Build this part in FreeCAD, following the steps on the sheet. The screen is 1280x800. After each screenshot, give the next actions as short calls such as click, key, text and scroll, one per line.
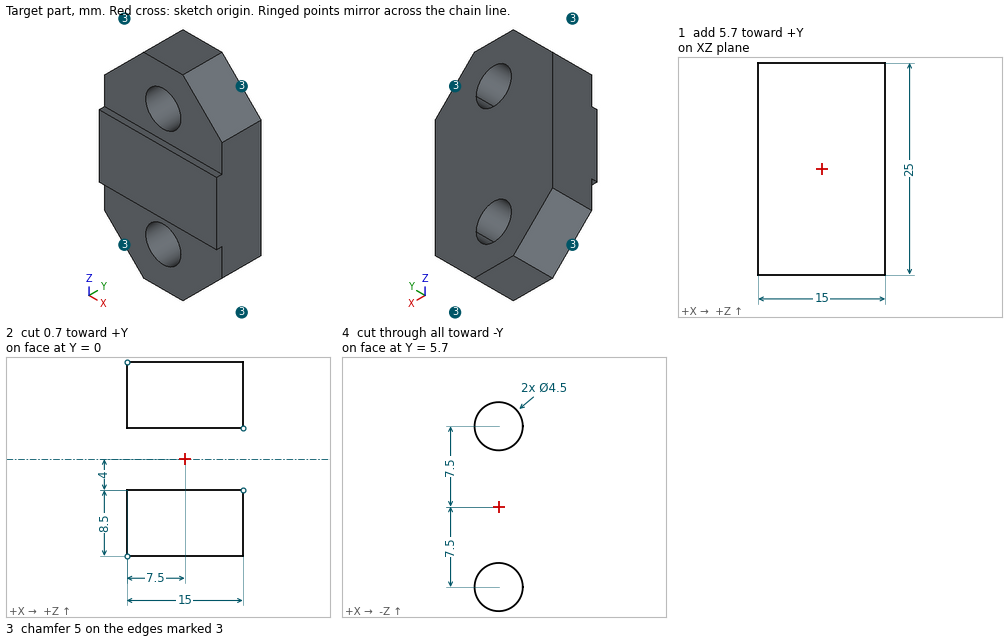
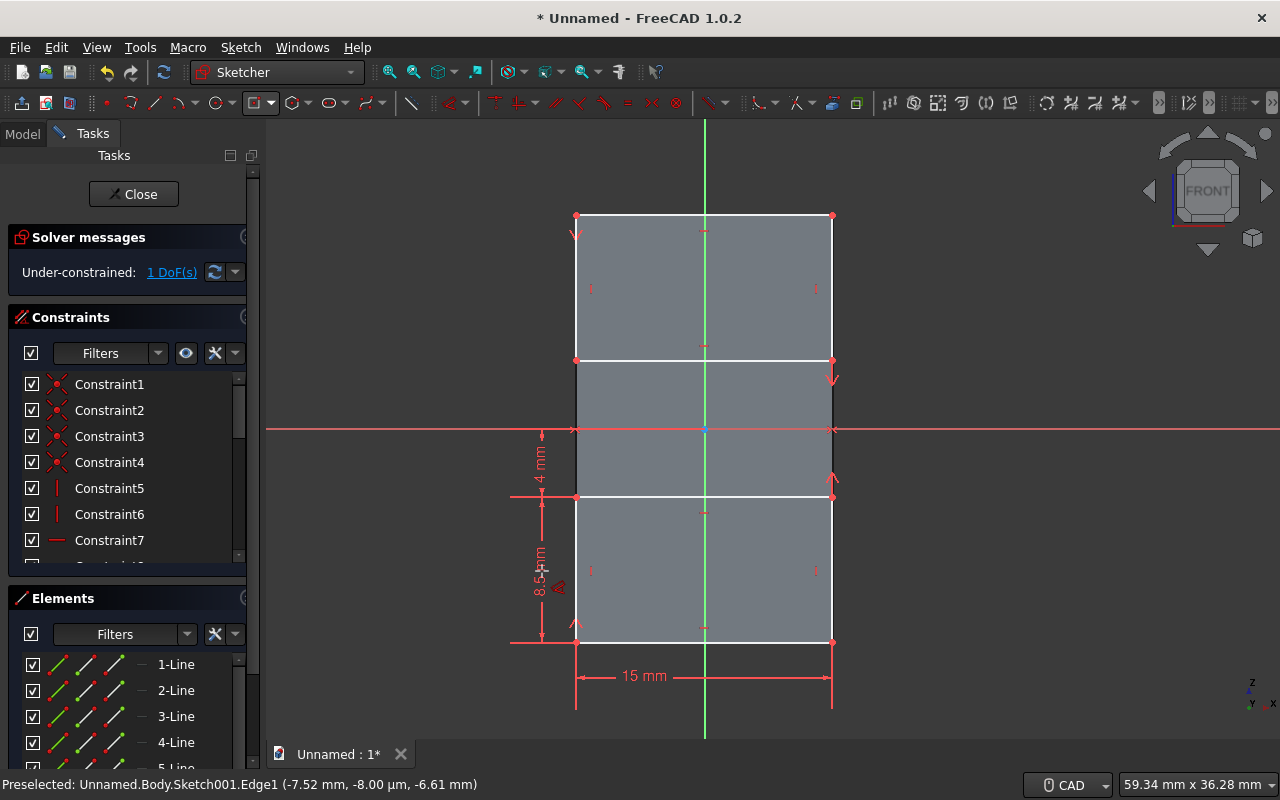
click(576, 497)
click(640, 531)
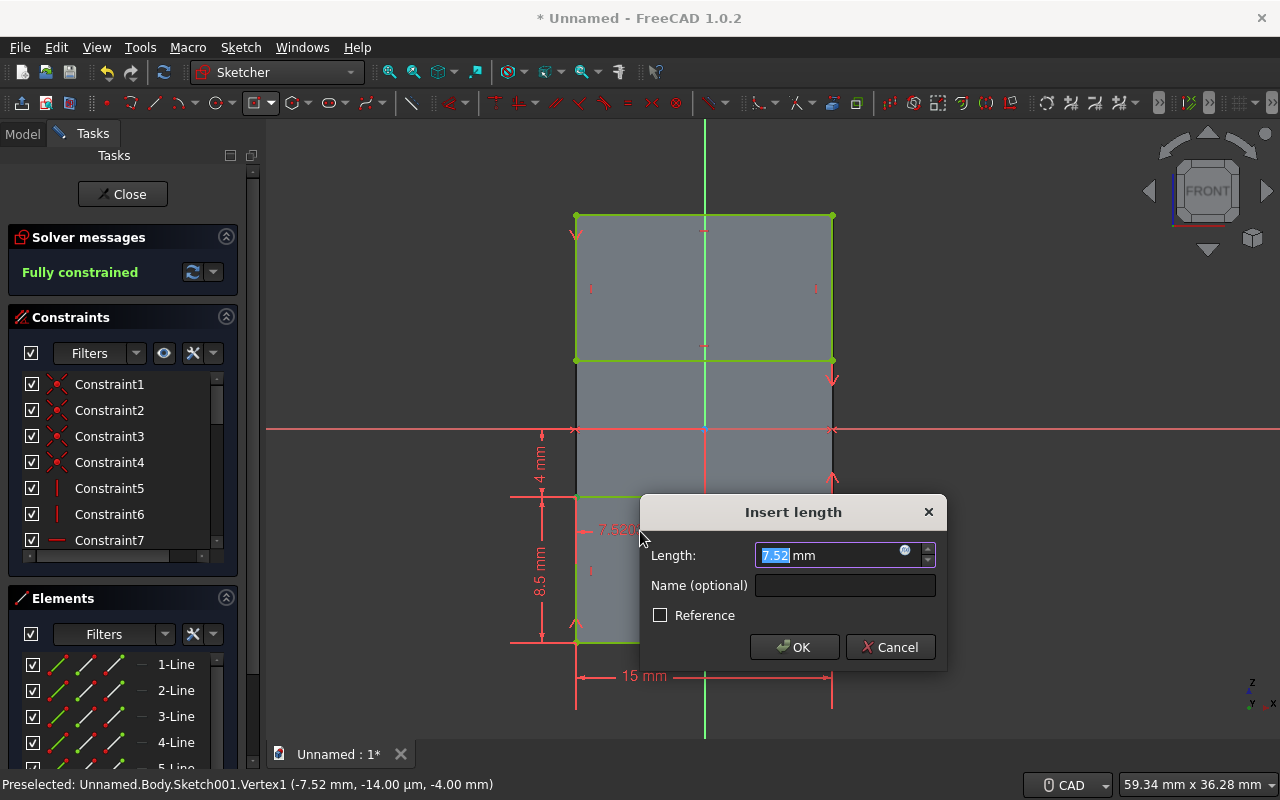
text(7.5)
key(Return)
key(Escape)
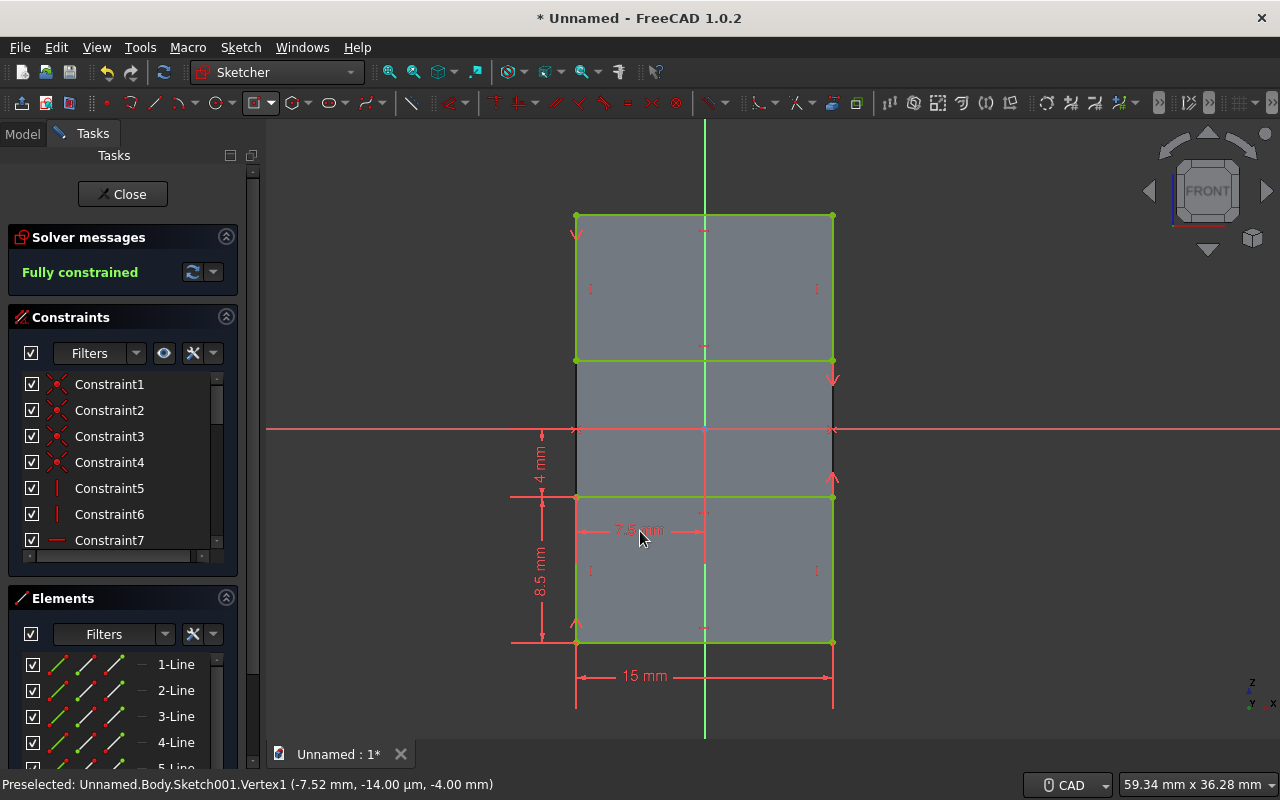
click(123, 194)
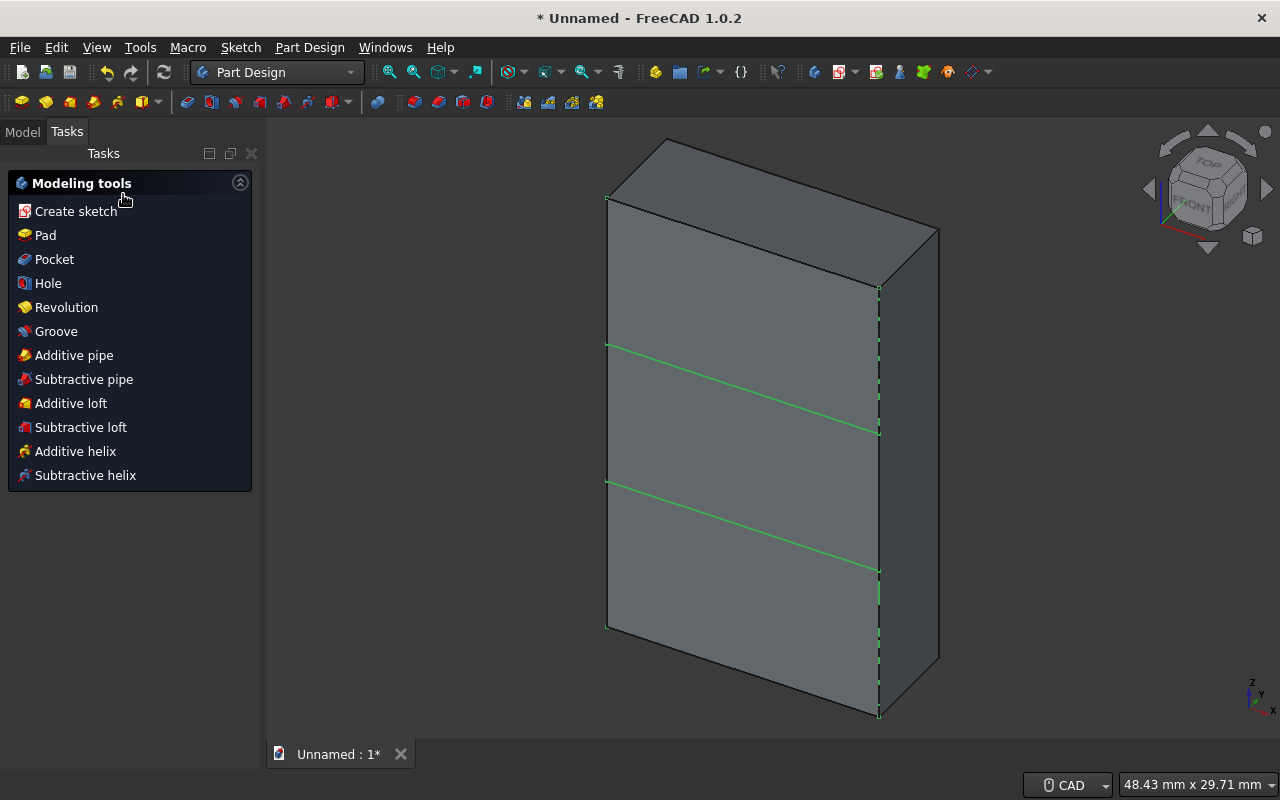
click(188, 102)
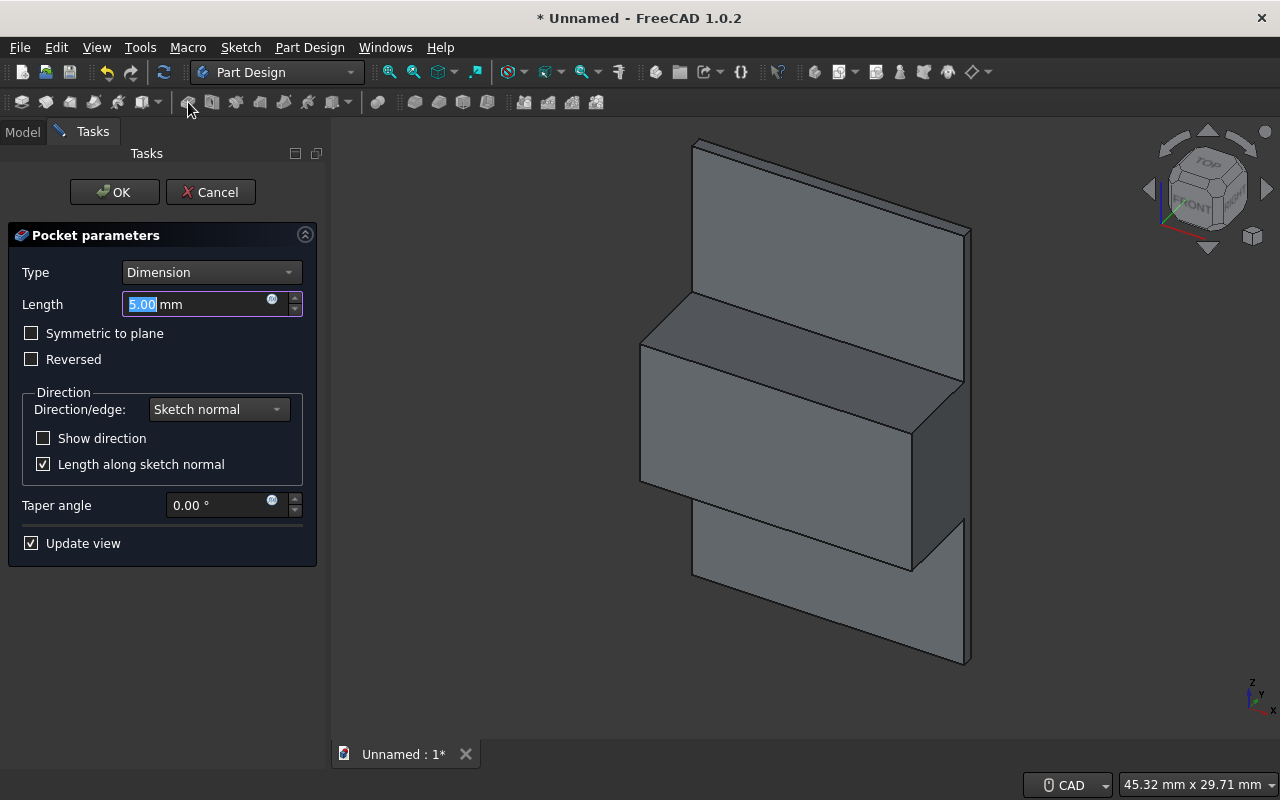
text(0.7)
key(Tab)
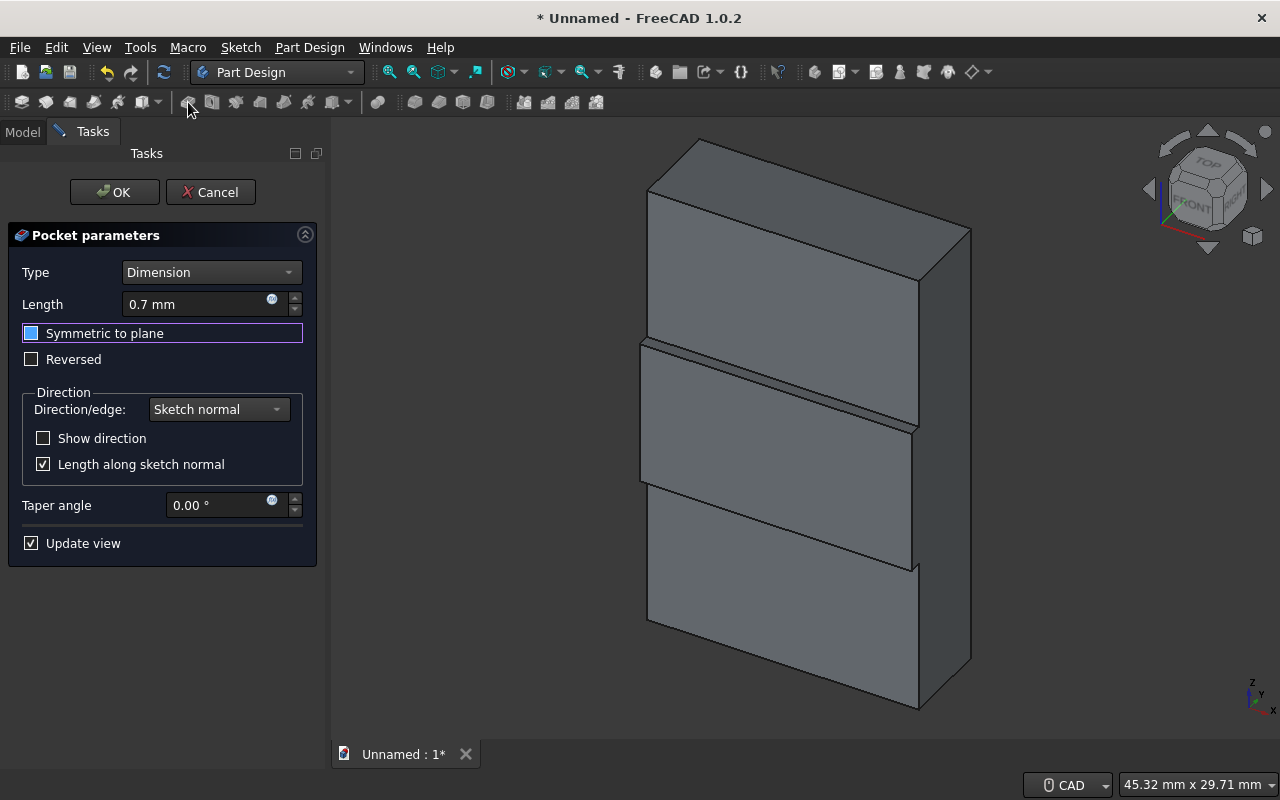
click(115, 192)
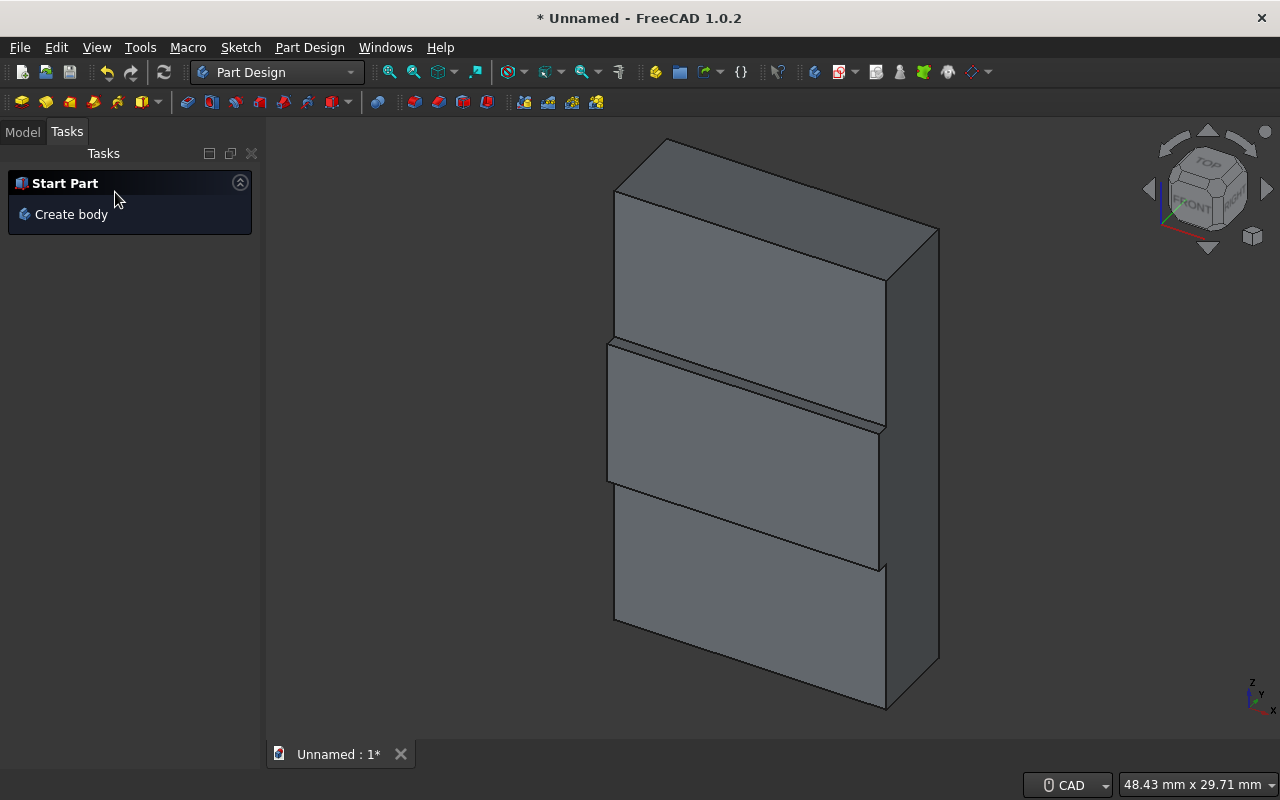
click(913, 254)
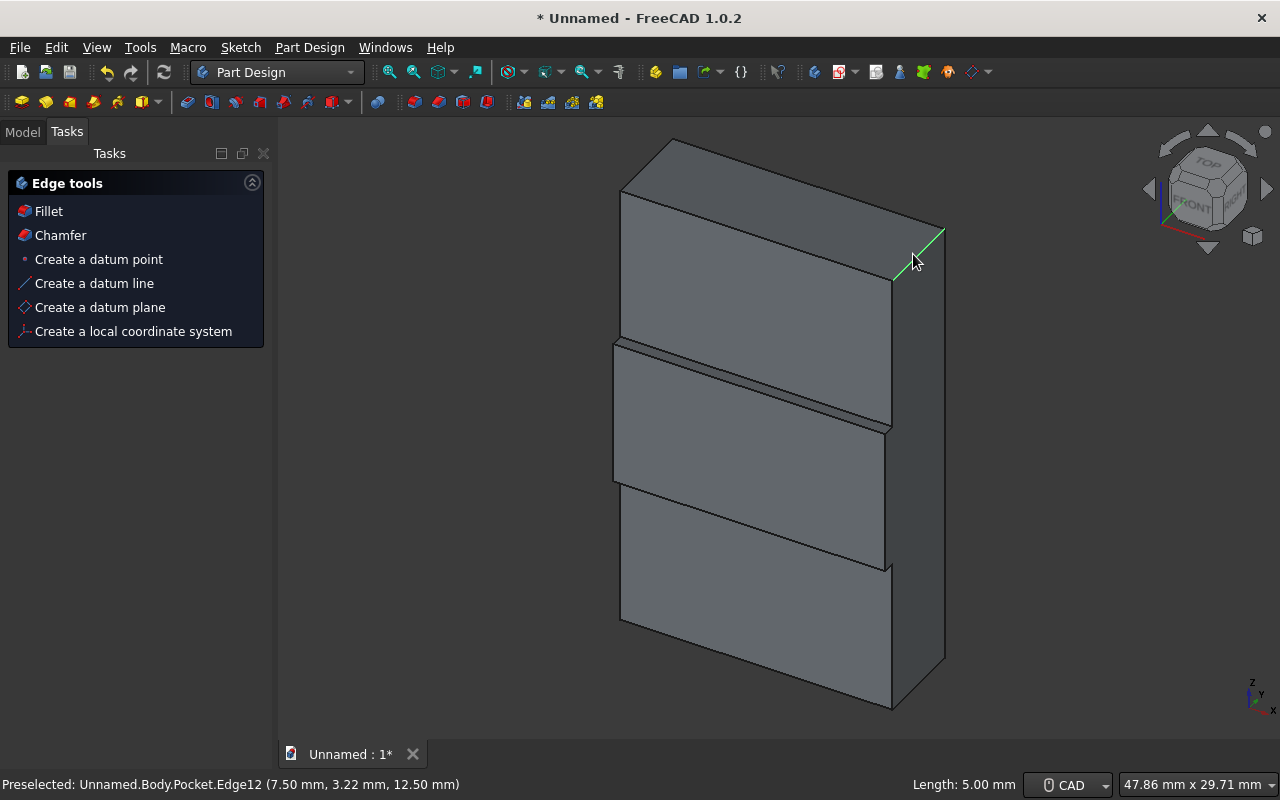
key(0)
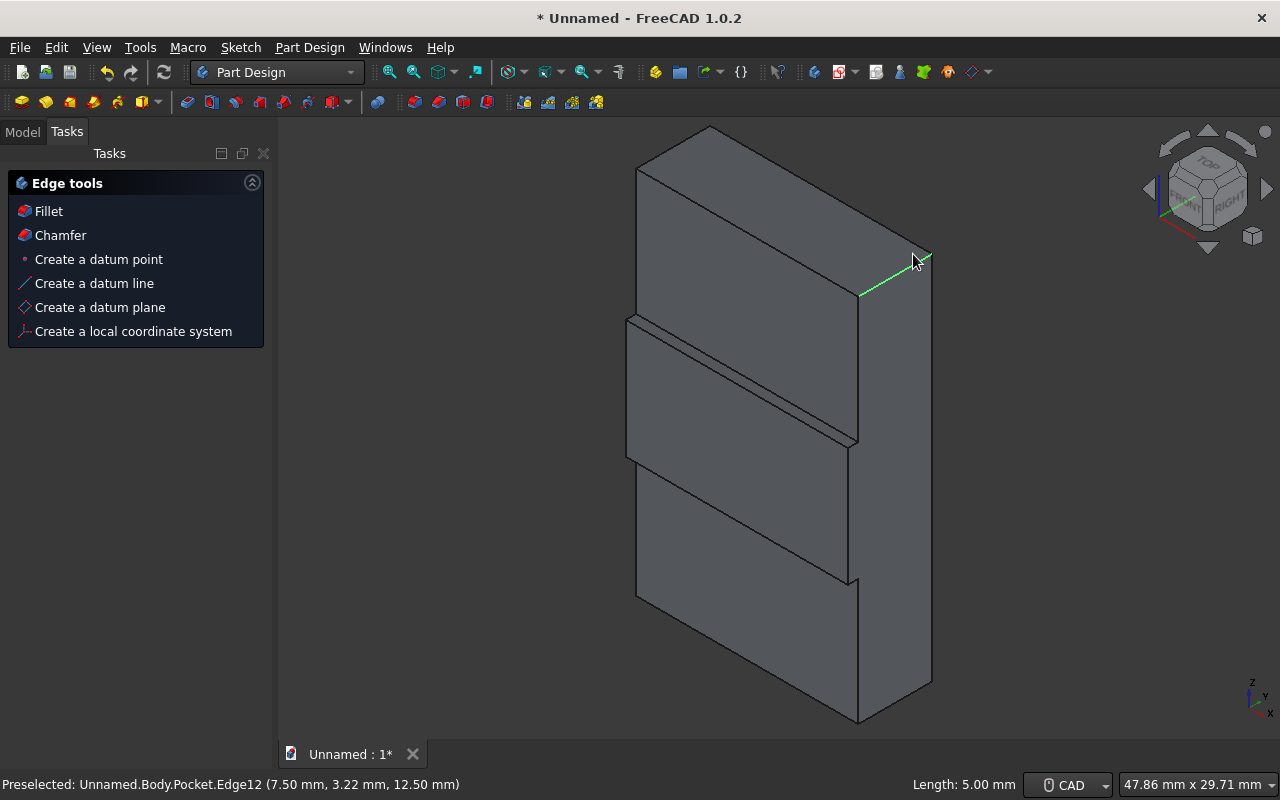
key(2)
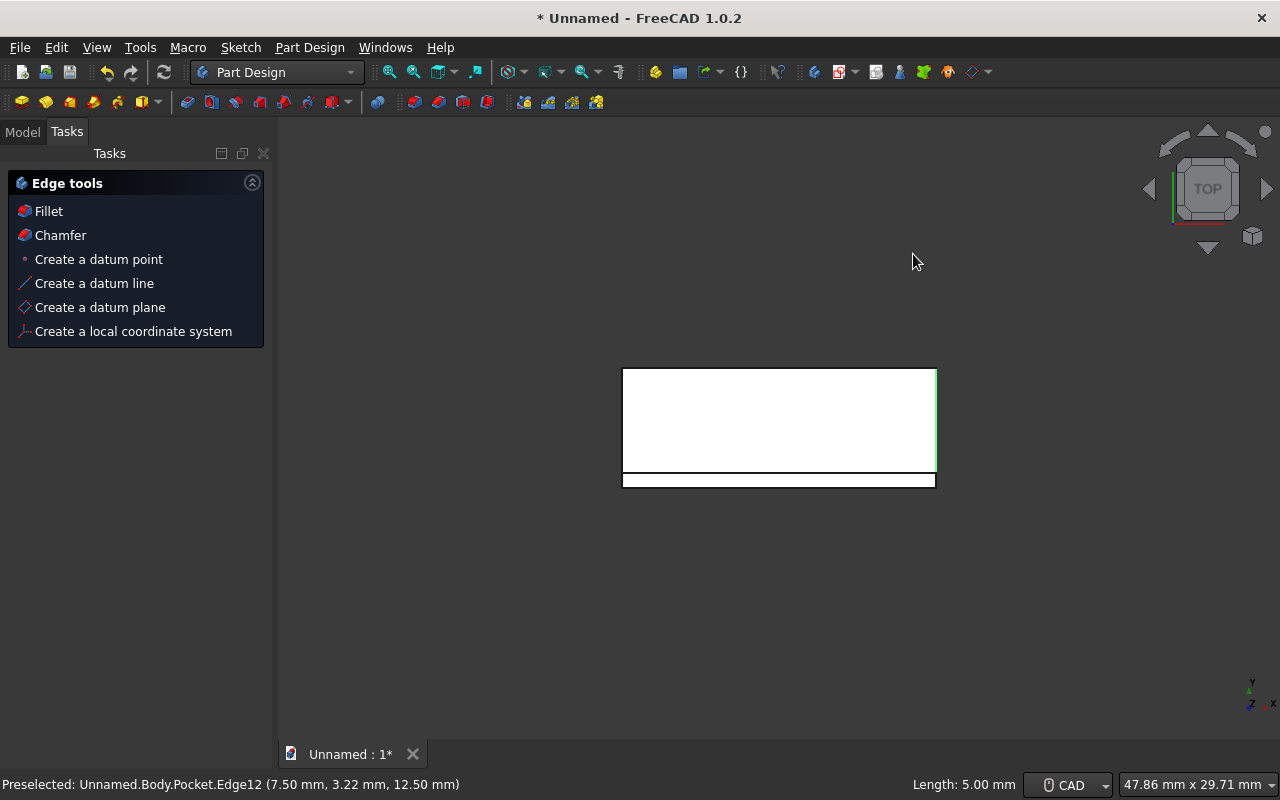
key(v)
key(f)